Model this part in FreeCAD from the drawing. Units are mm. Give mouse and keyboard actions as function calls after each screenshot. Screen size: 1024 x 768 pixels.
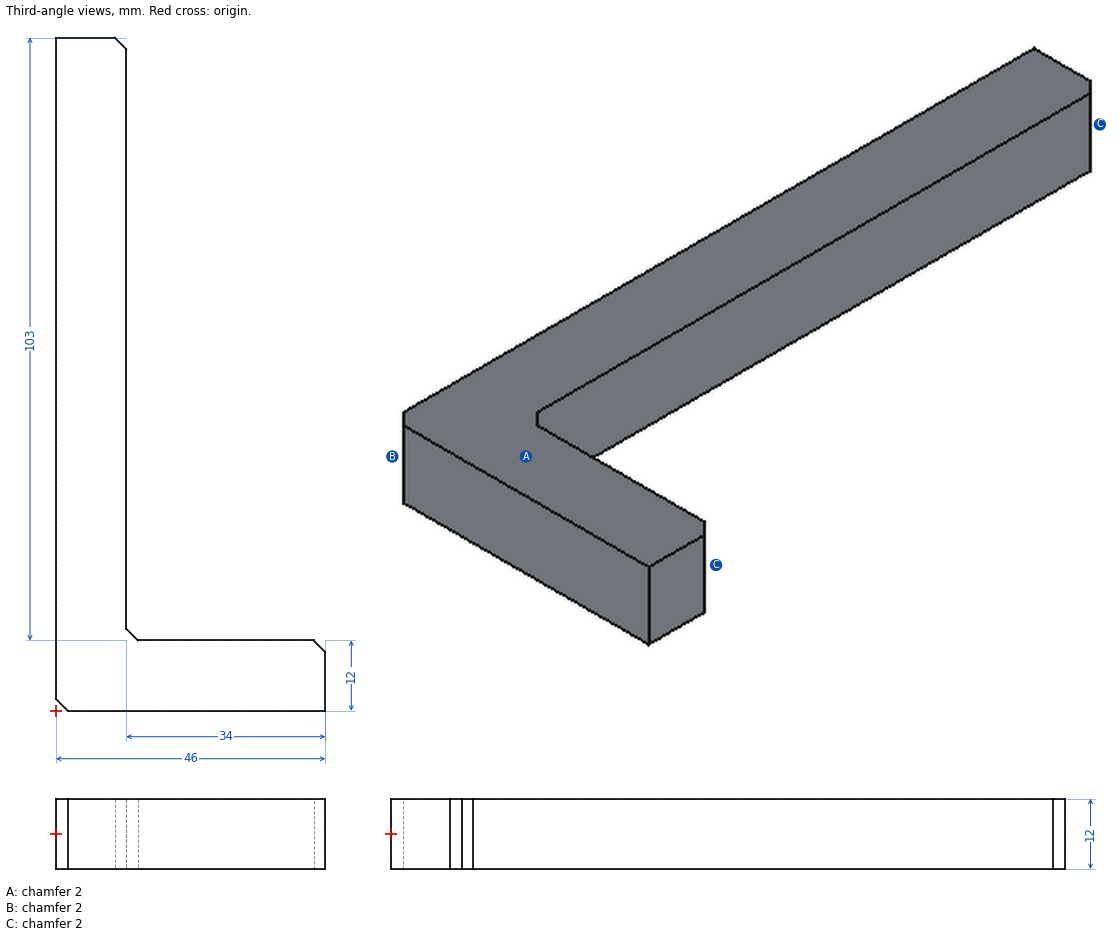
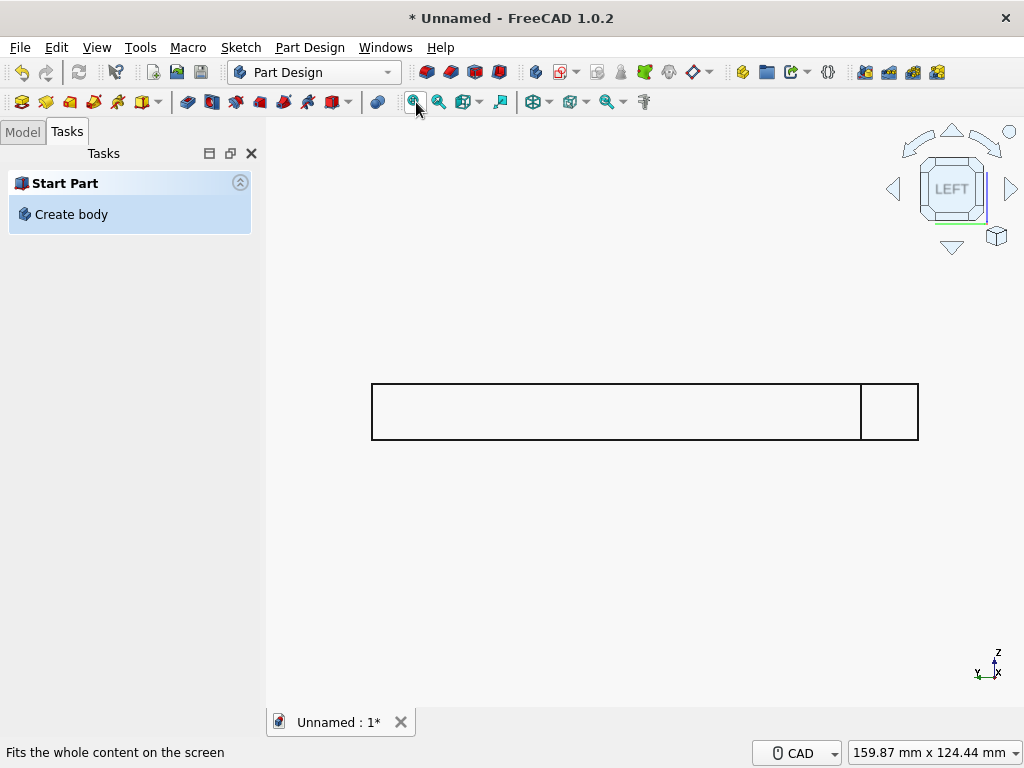
key(0)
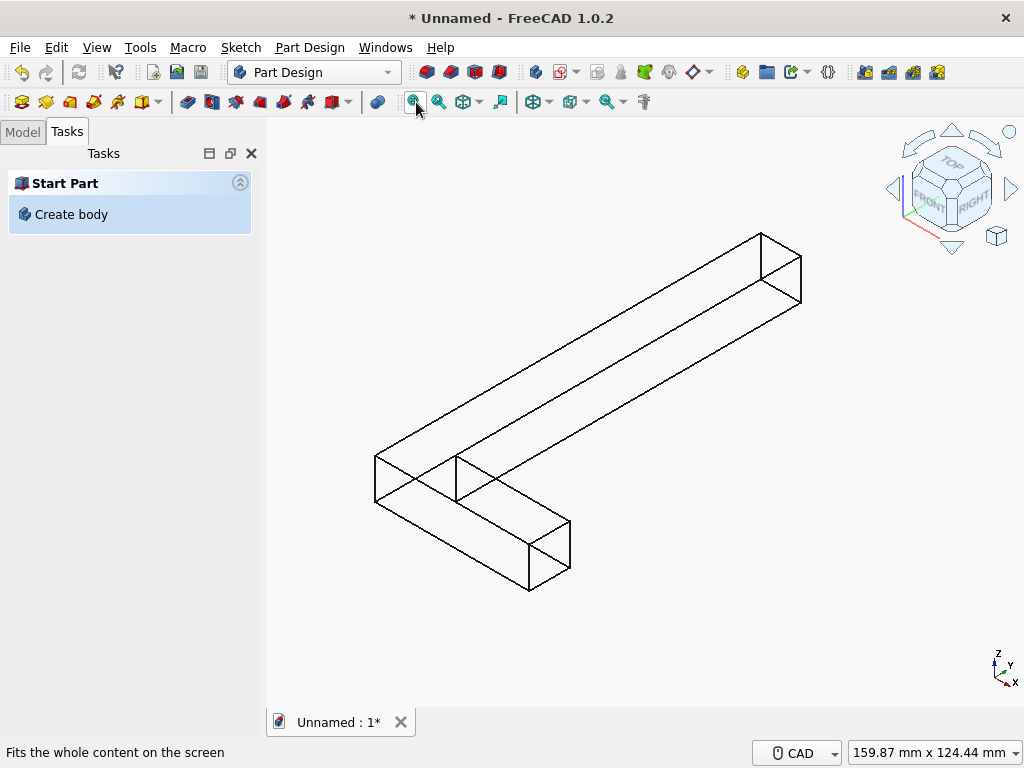
click(456, 478)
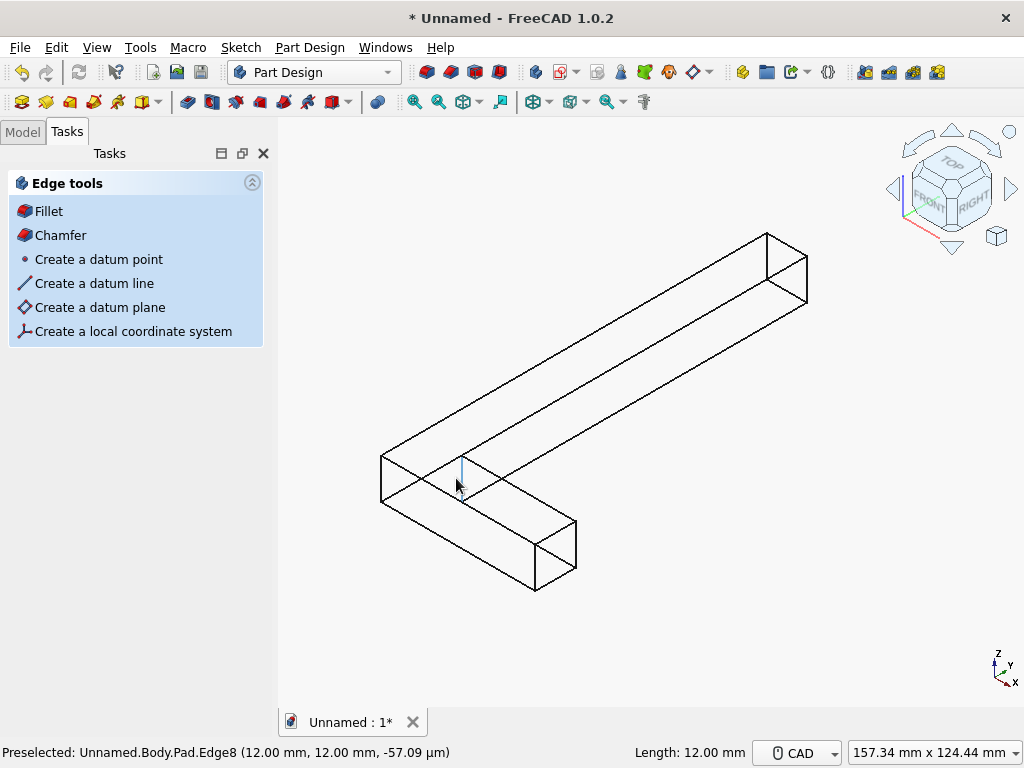
key(v)
key(1)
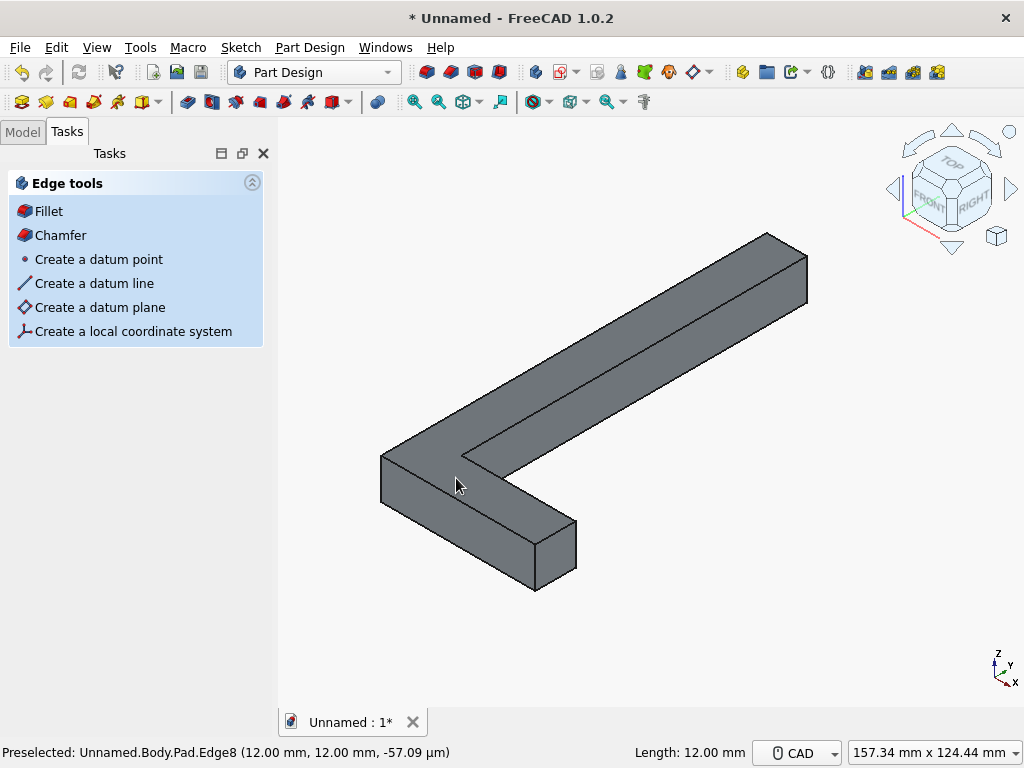
click(452, 72)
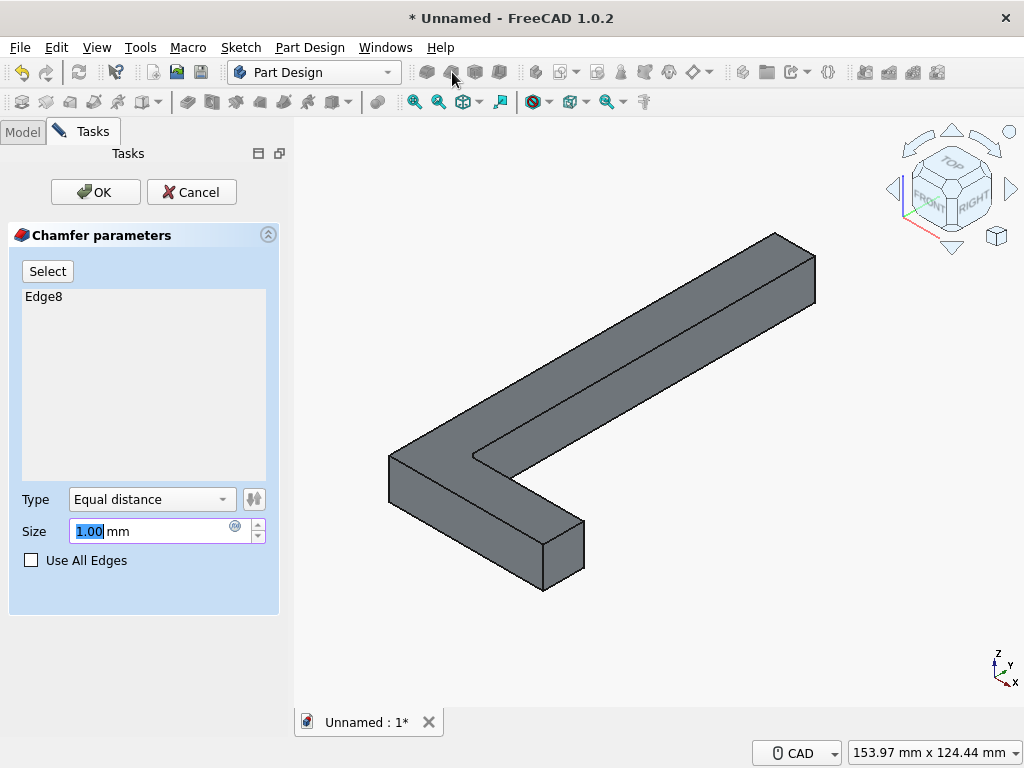
text(2)
key(Tab)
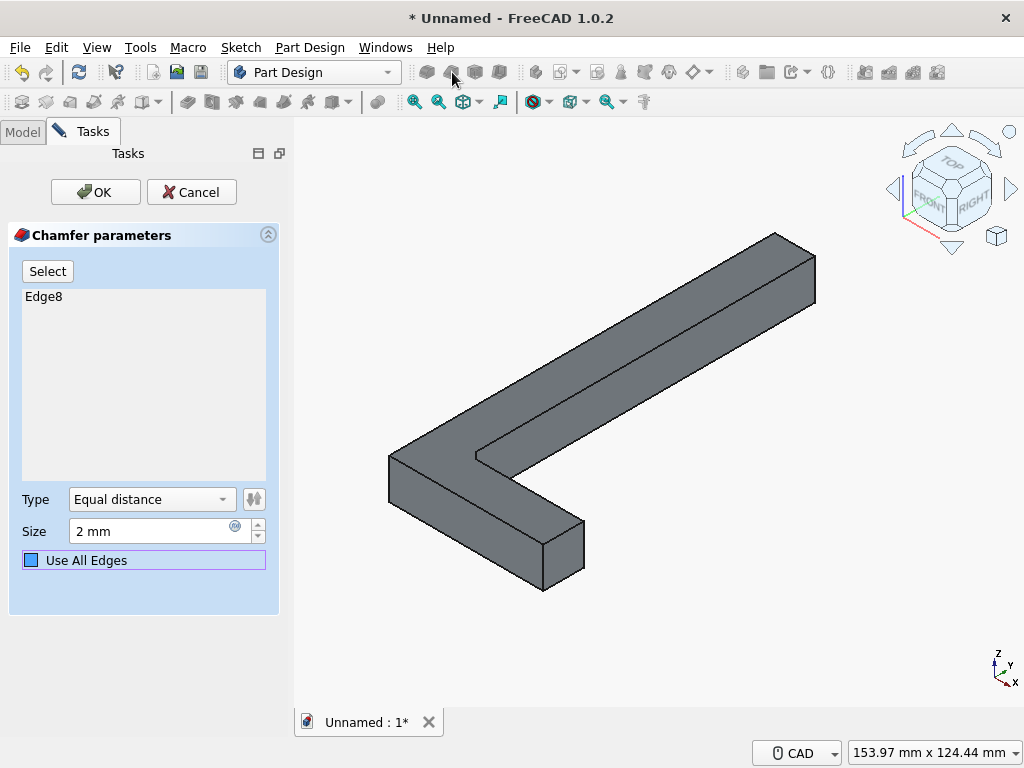
click(96, 192)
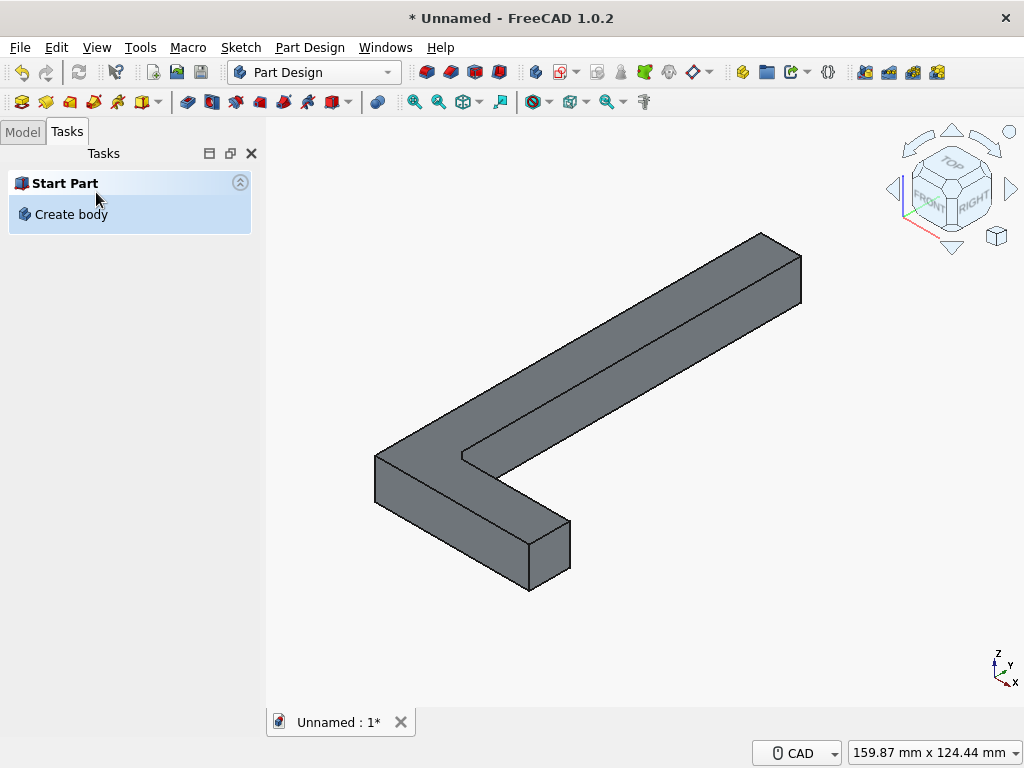
key(2)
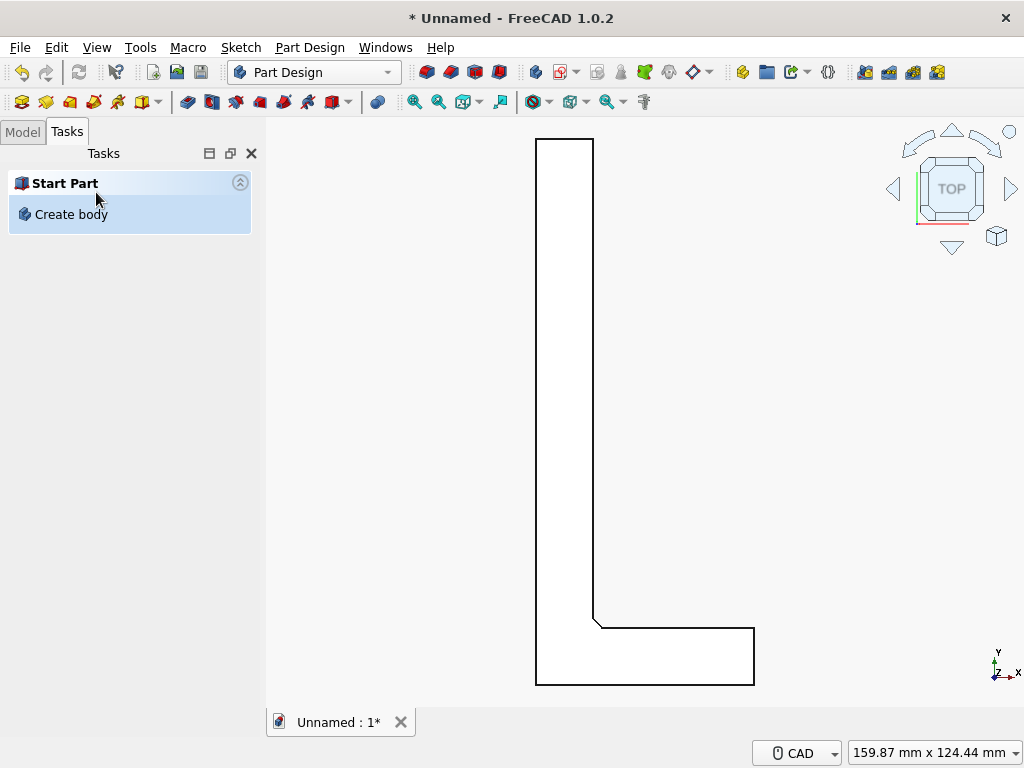
key(0)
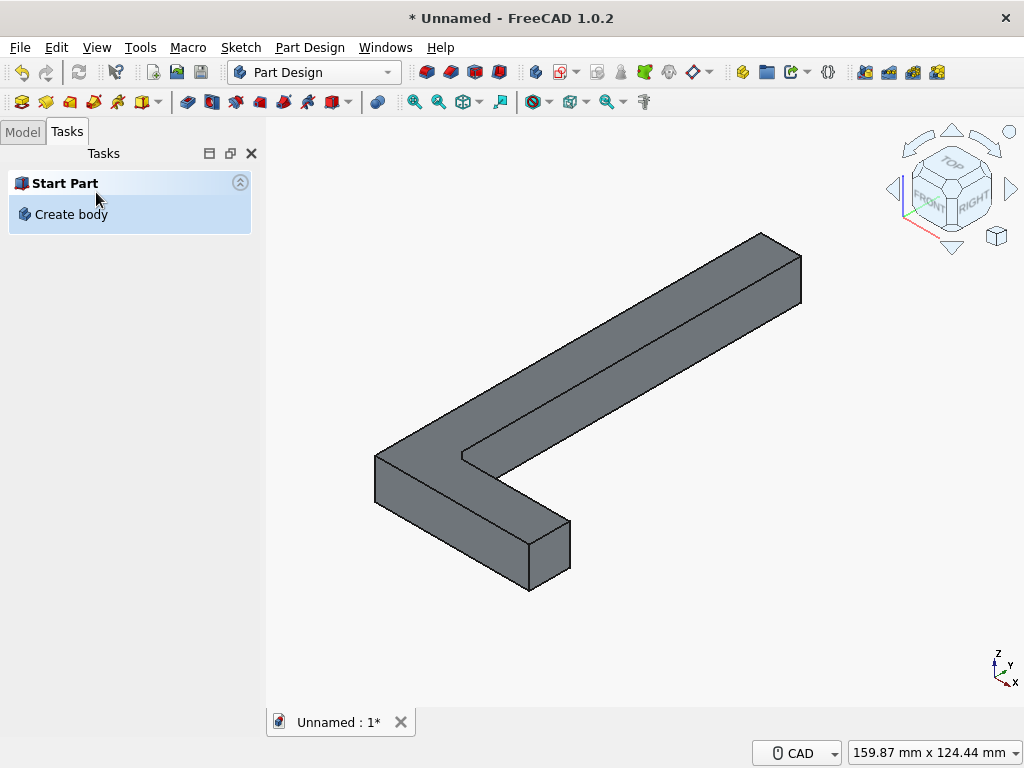
key(1)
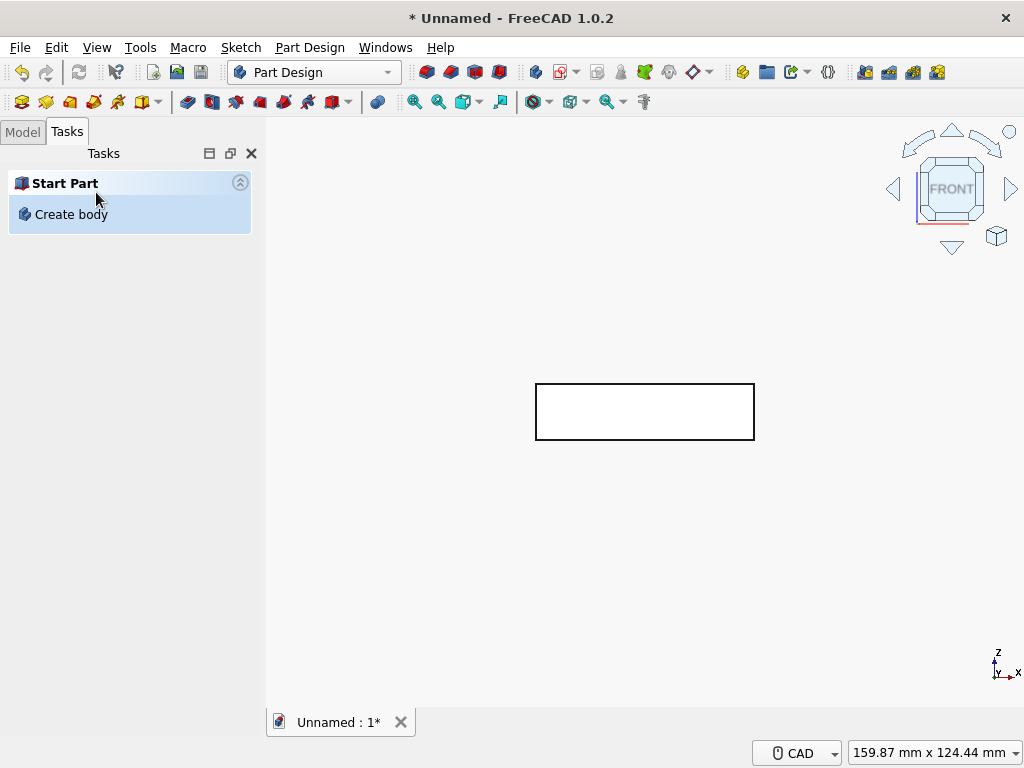
click(416, 102)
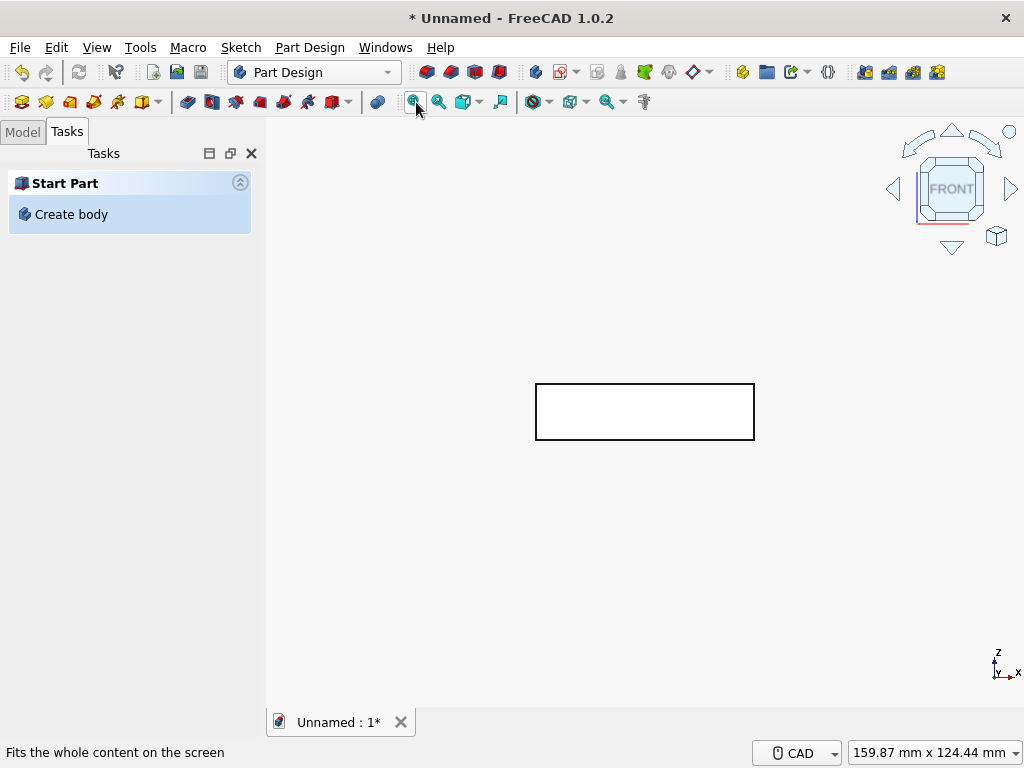
click(536, 411)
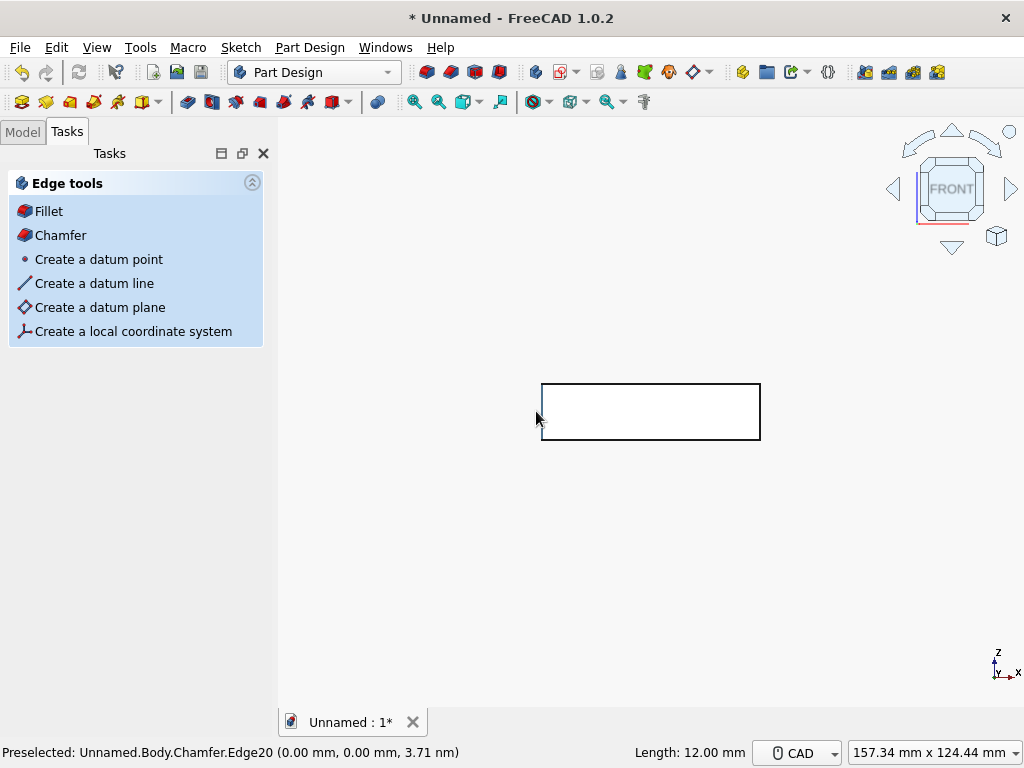
click(452, 72)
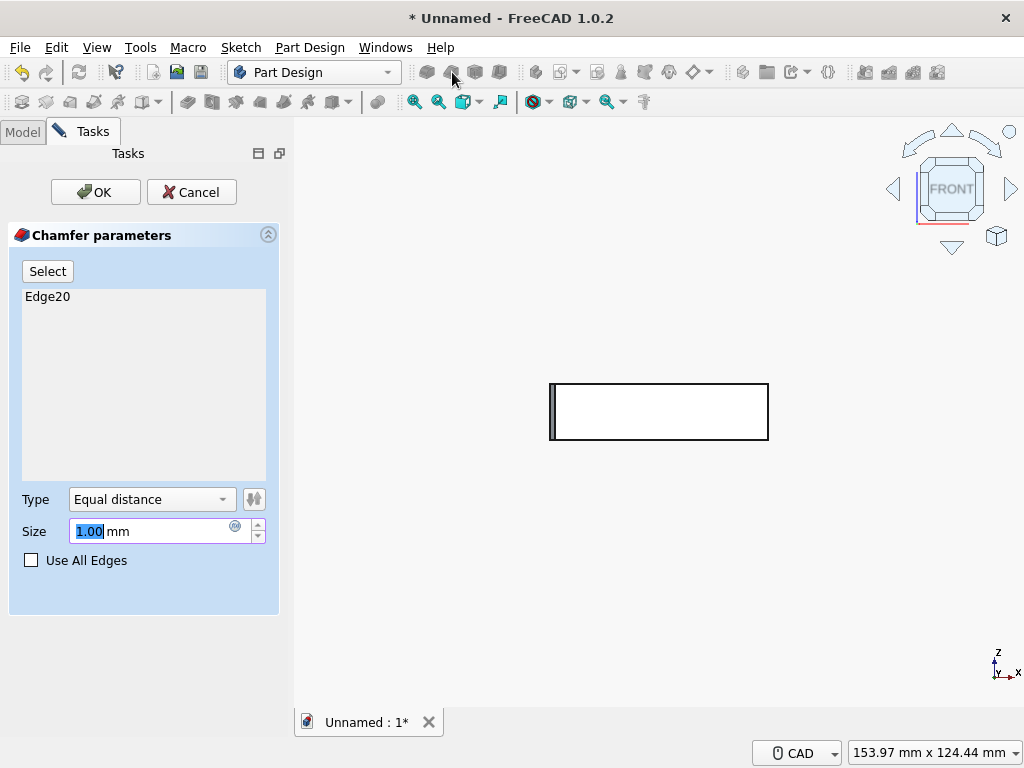
text(2)
key(Tab)